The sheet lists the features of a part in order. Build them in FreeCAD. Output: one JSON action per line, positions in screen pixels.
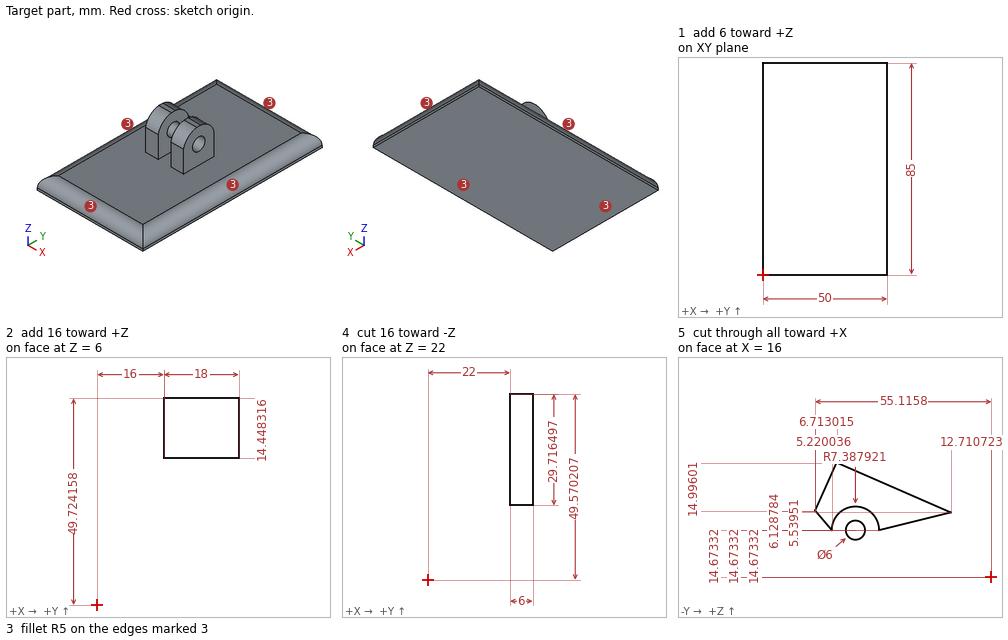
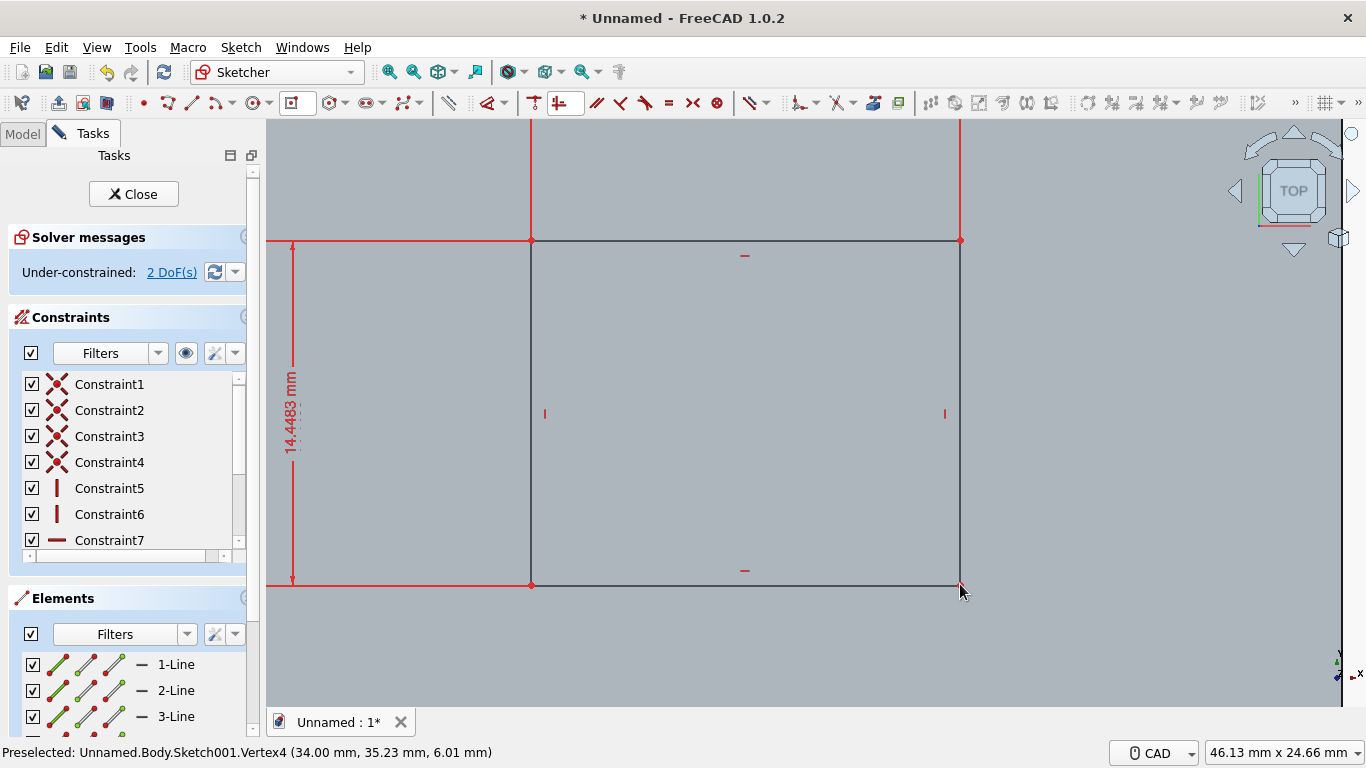
{"action": "left_click", "coordinate": [488, 104]}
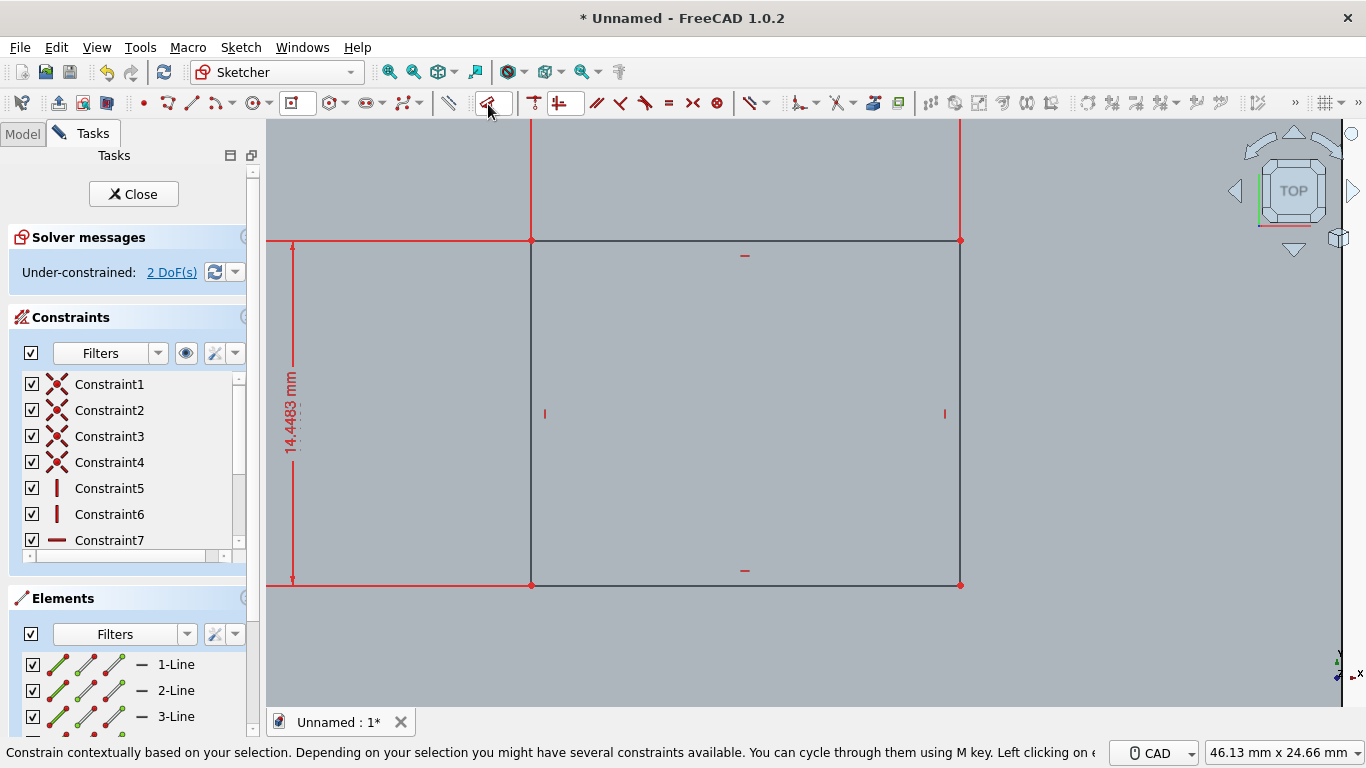
{"action": "left_click", "coordinate": [531, 241]}
{"action": "left_click", "coordinate": [413, 207]}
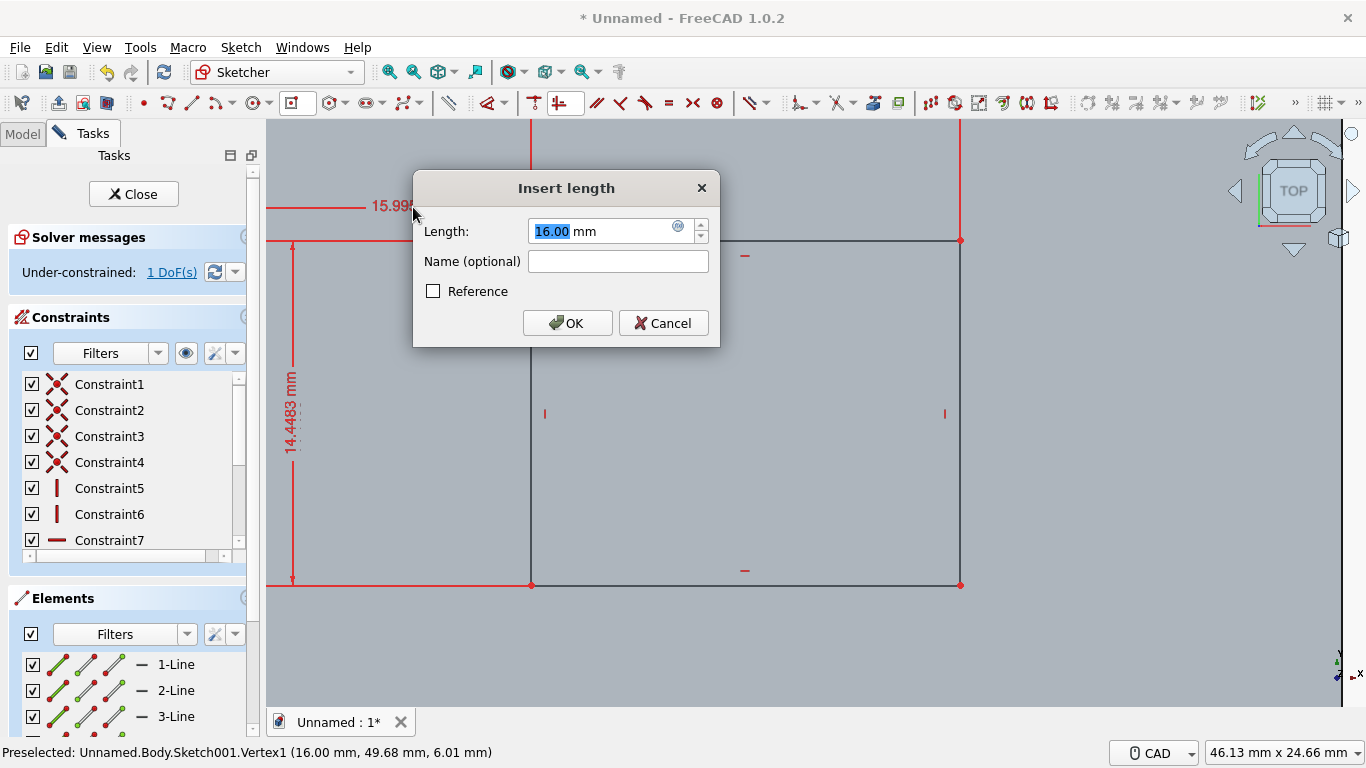
{"action": "type", "text": "16"}
{"action": "key", "text": "Return"}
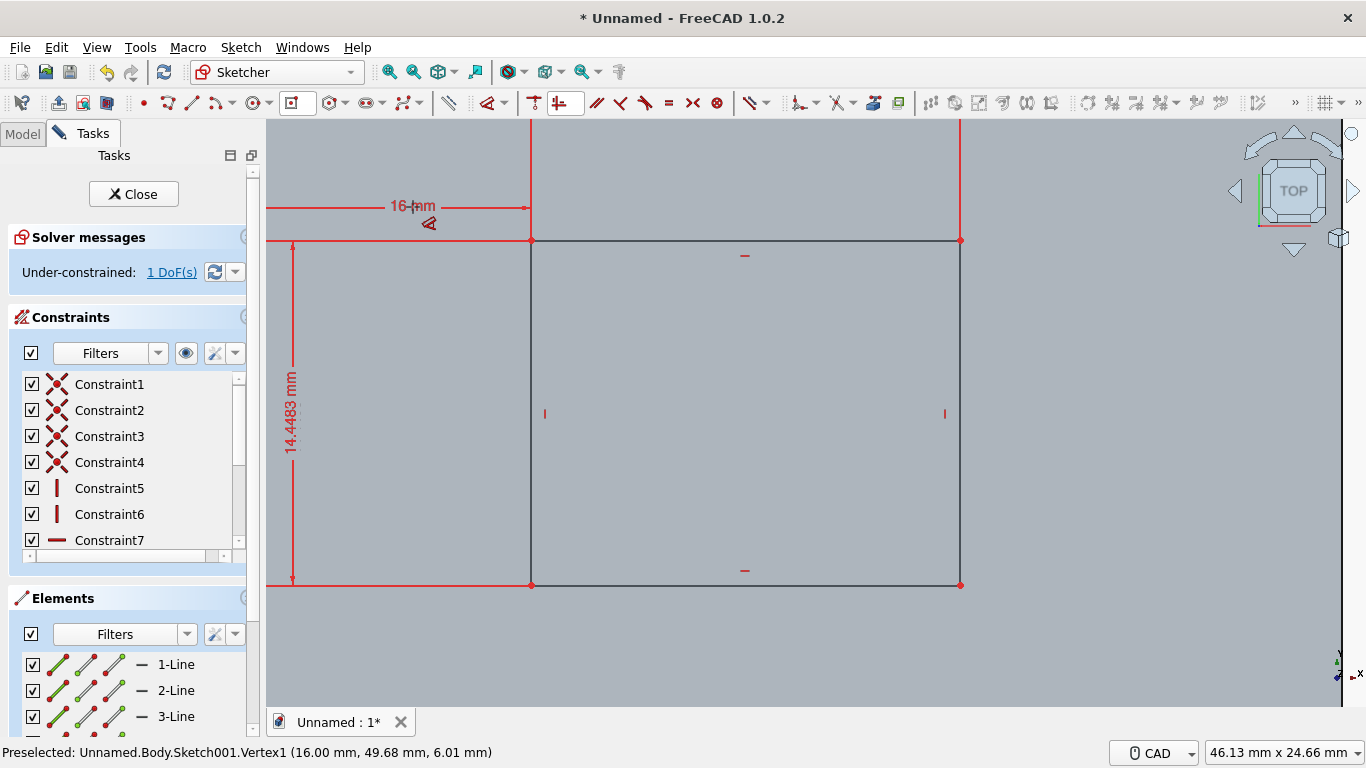
{"action": "left_click", "coordinate": [531, 241]}
{"action": "left_click", "coordinate": [565, 460]}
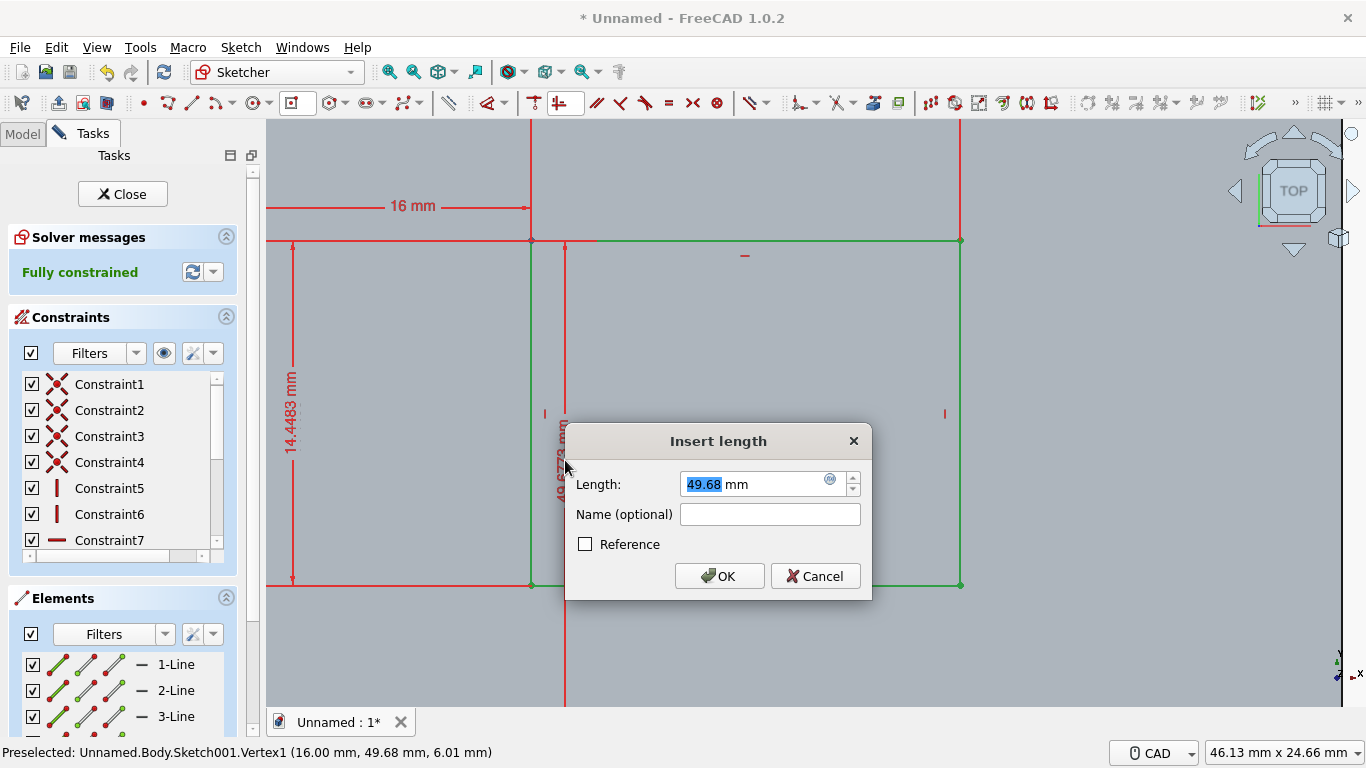
{"action": "type", "text": "49.724158"}
{"action": "key", "text": "Return"}
{"action": "key", "text": "Escape"}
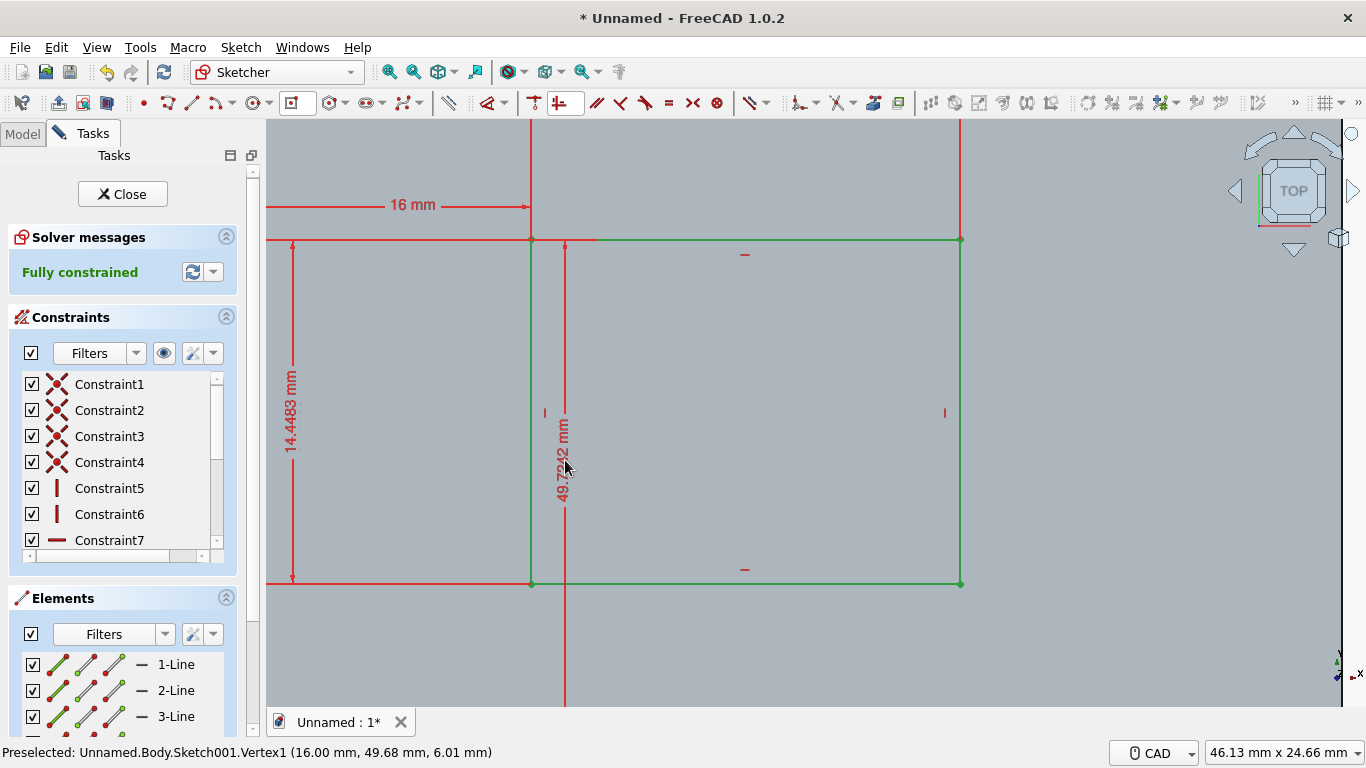
{"action": "left_click", "coordinate": [123, 194]}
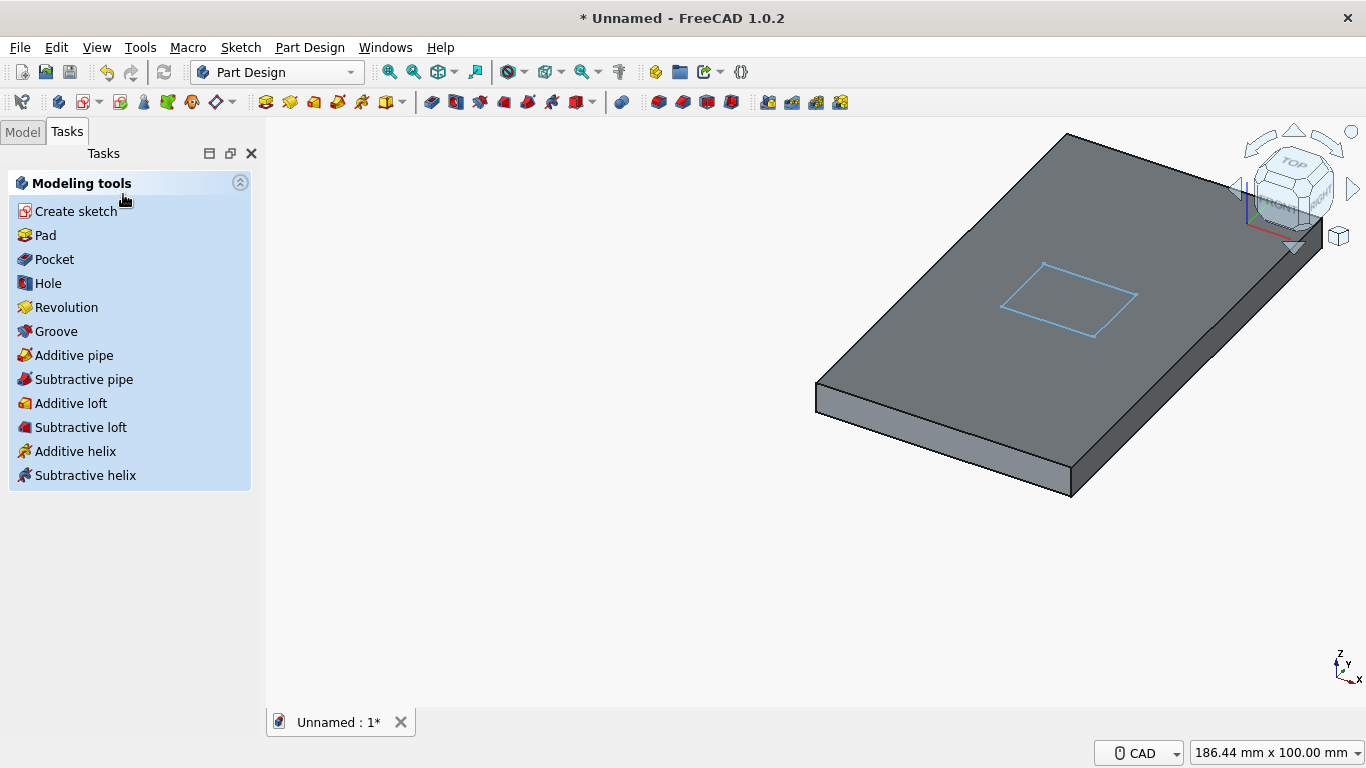
{"action": "left_click", "coordinate": [266, 102]}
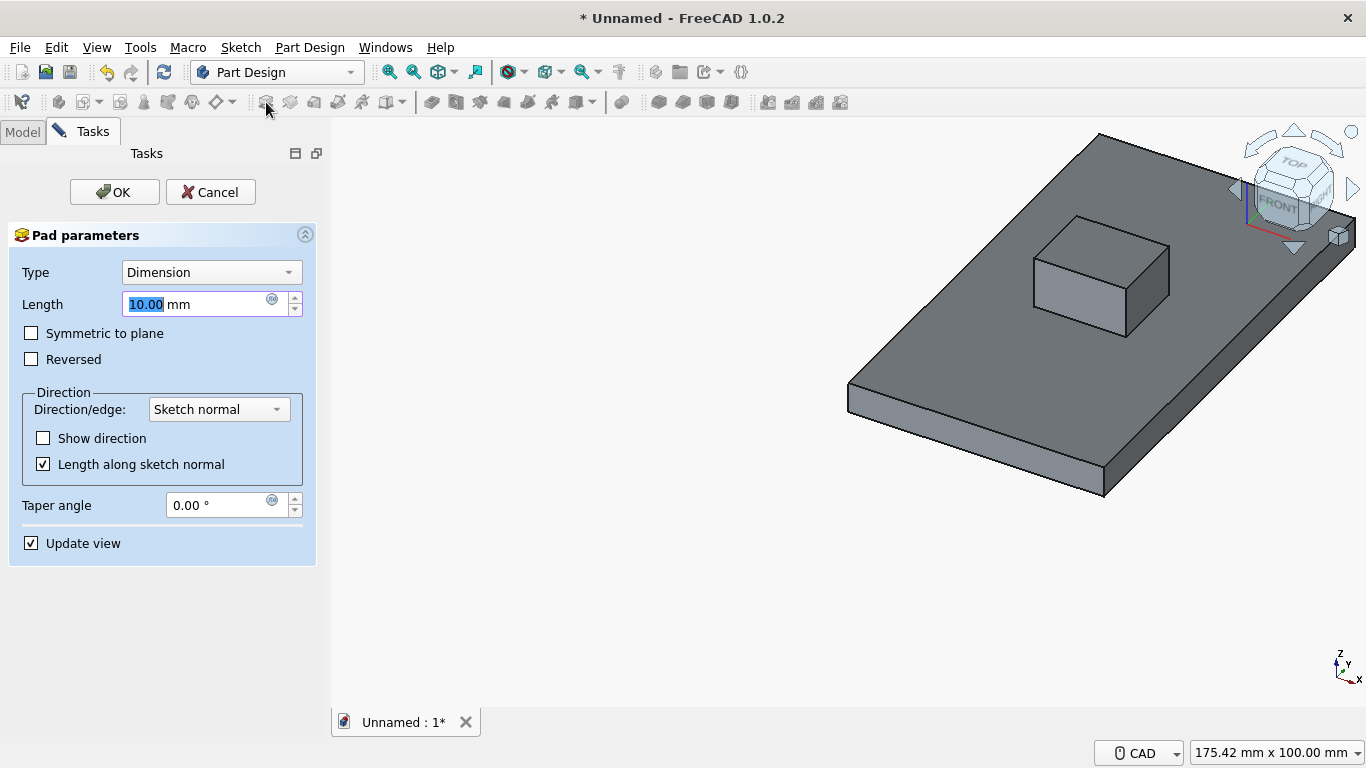
{"action": "type", "text": "16"}
{"action": "key", "text": "Tab"}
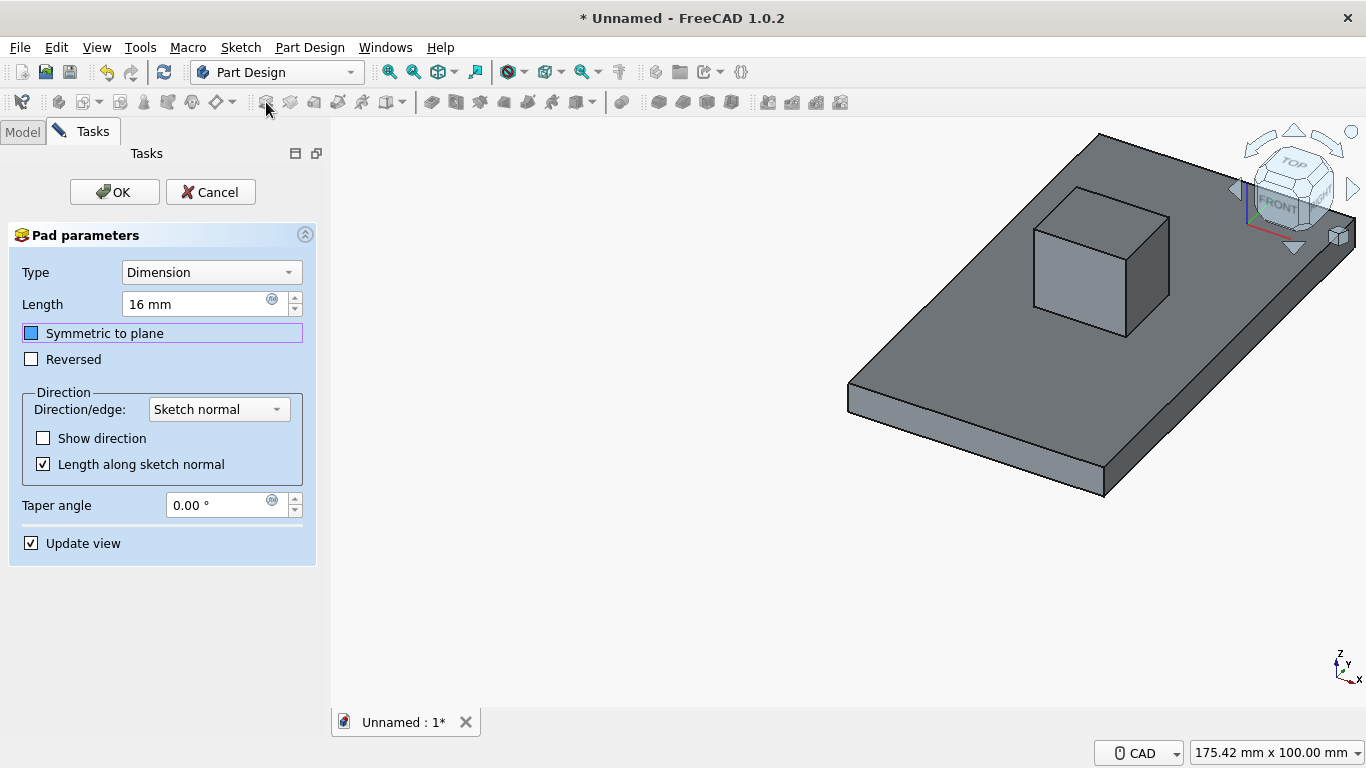
{"action": "left_click", "coordinate": [115, 192]}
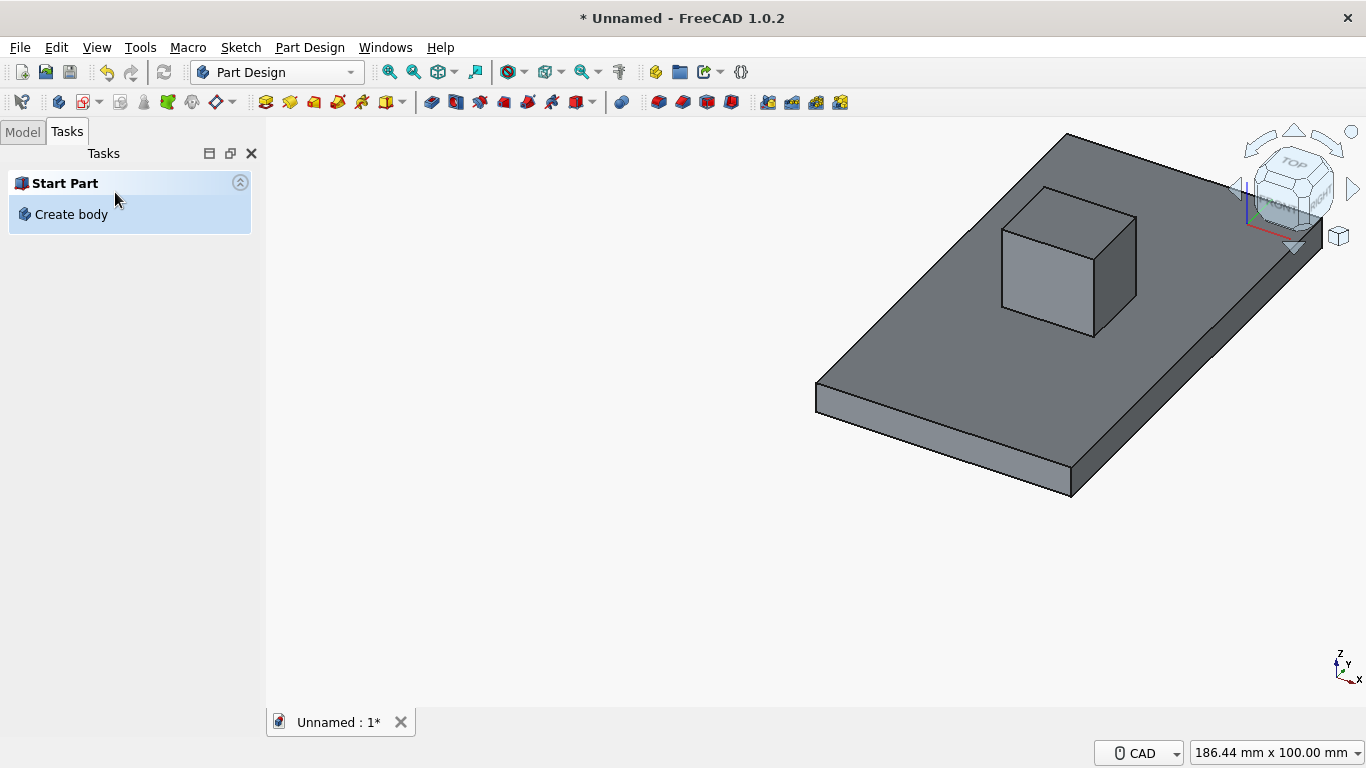
{"action": "key", "text": "v f"}